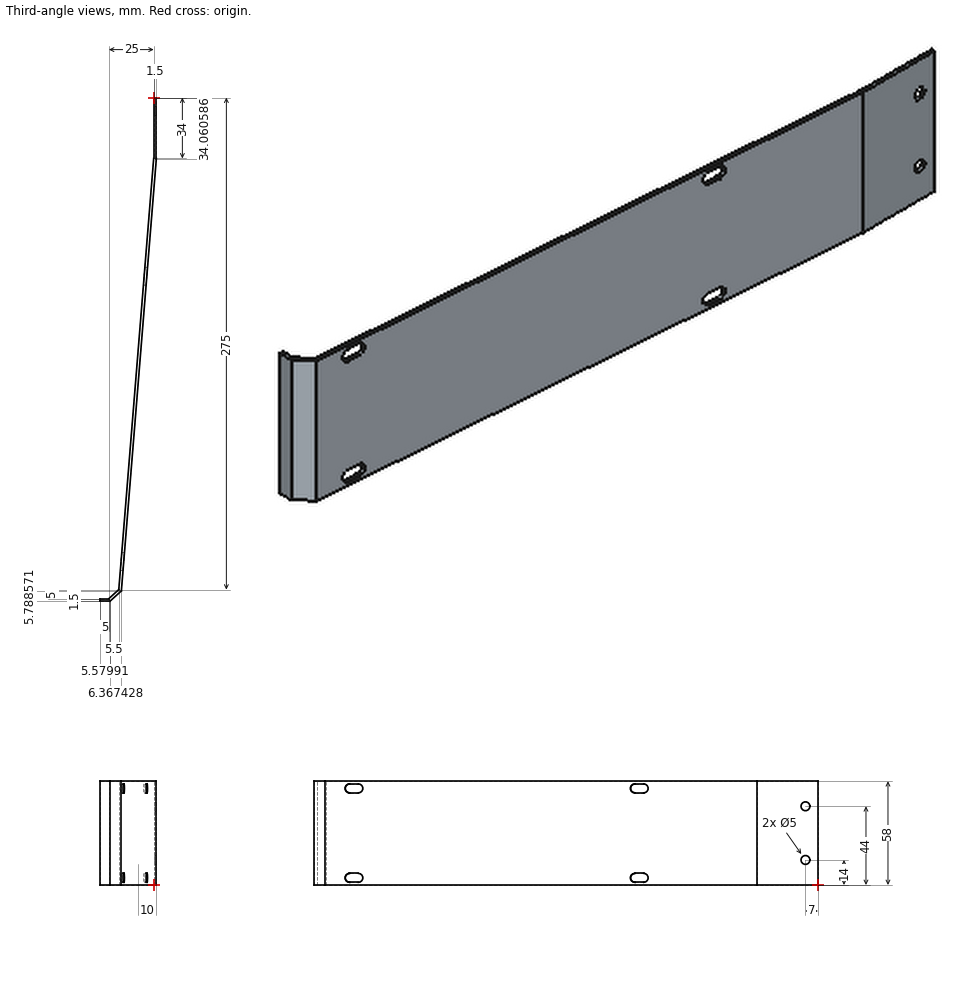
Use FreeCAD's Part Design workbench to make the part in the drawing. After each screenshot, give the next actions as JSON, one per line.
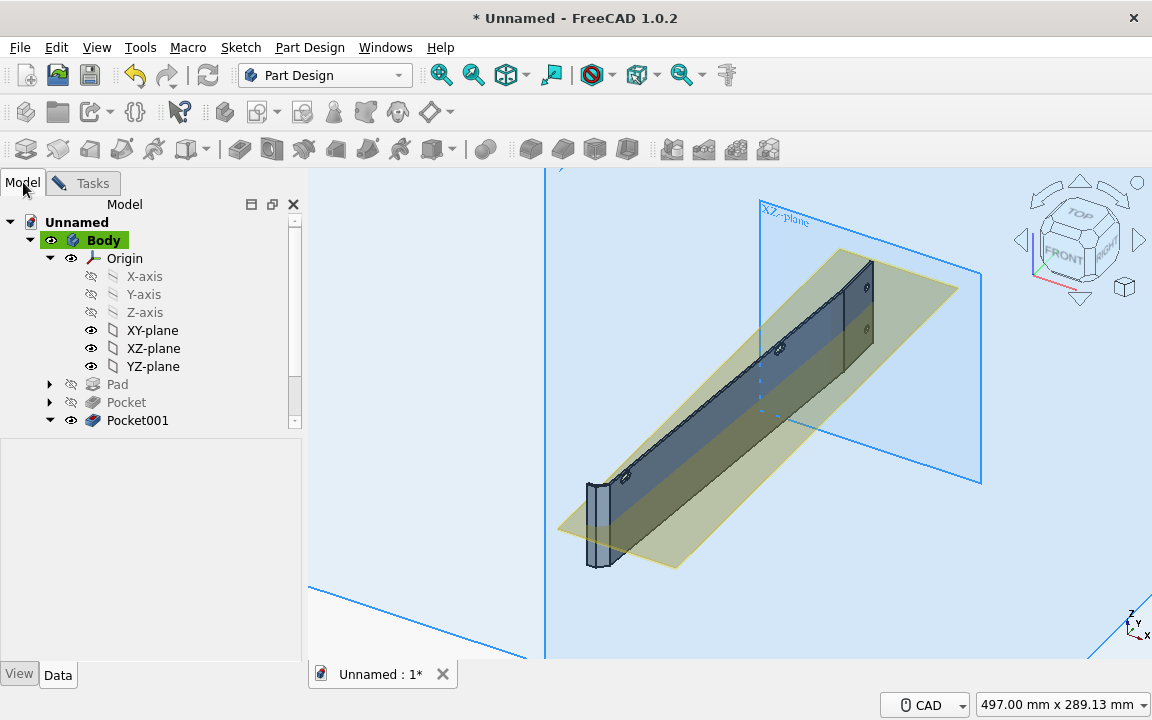
{"action": "scroll", "coordinate": [100, 326], "scroll_direction": "down", "scroll_amount": 3}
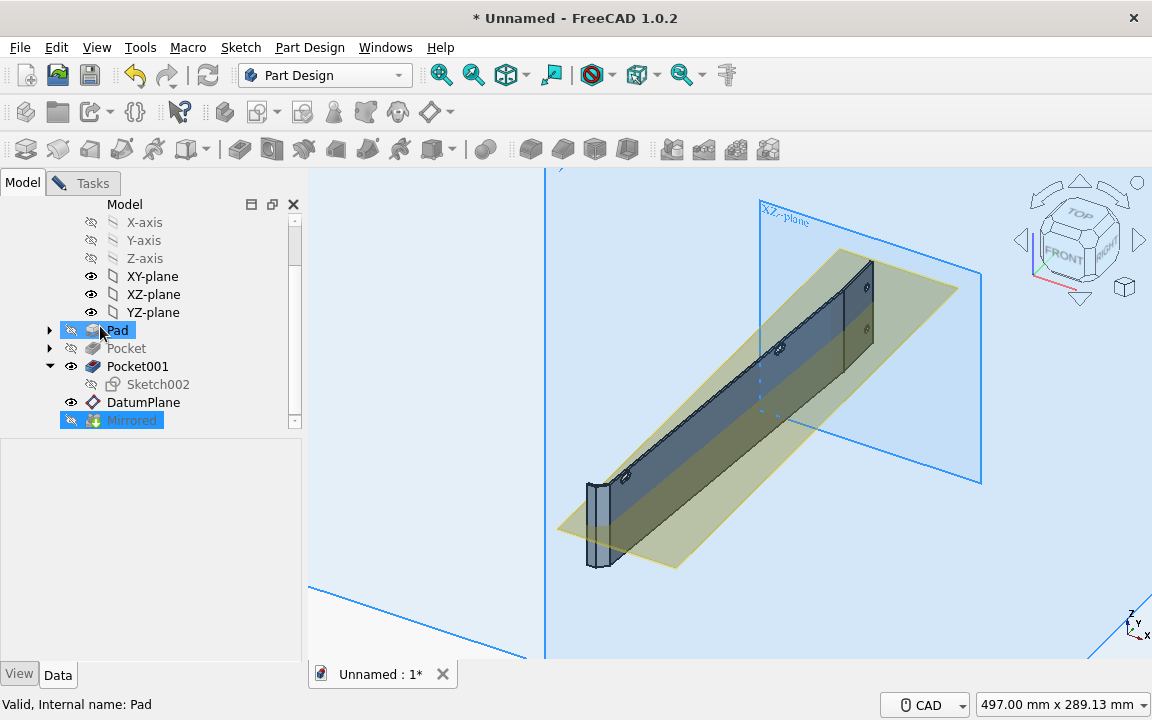
{"action": "left_click", "coordinate": [116, 402]}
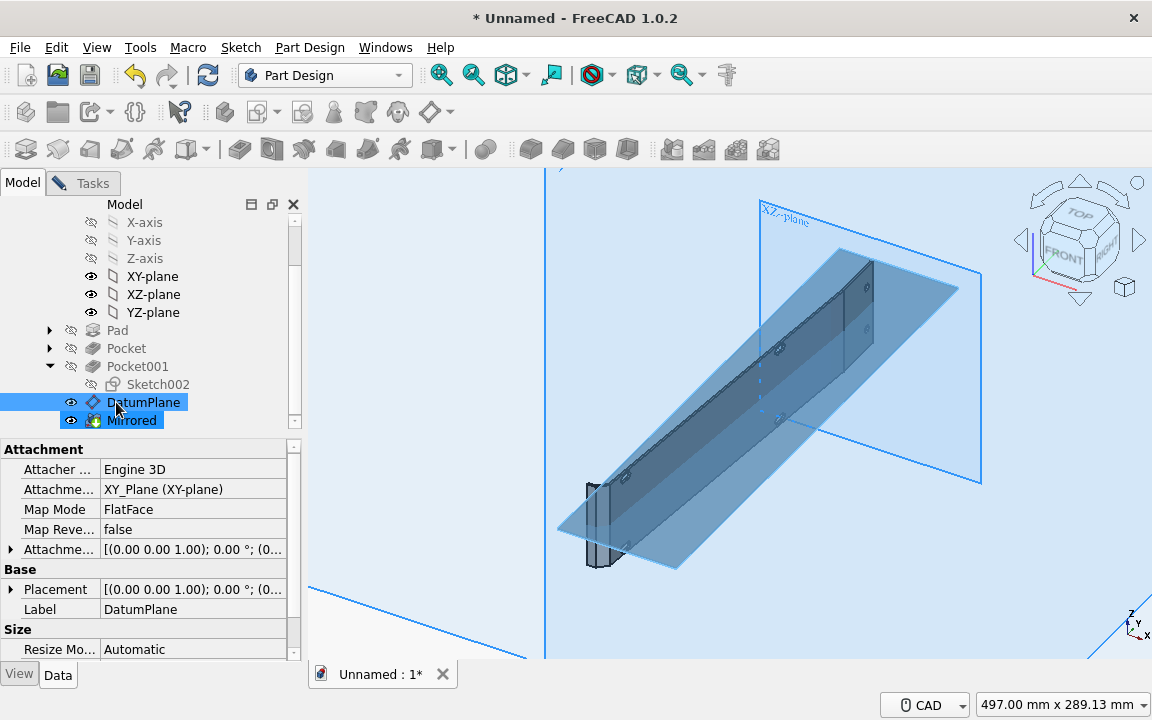
{"action": "left_click", "coordinate": [84, 182]}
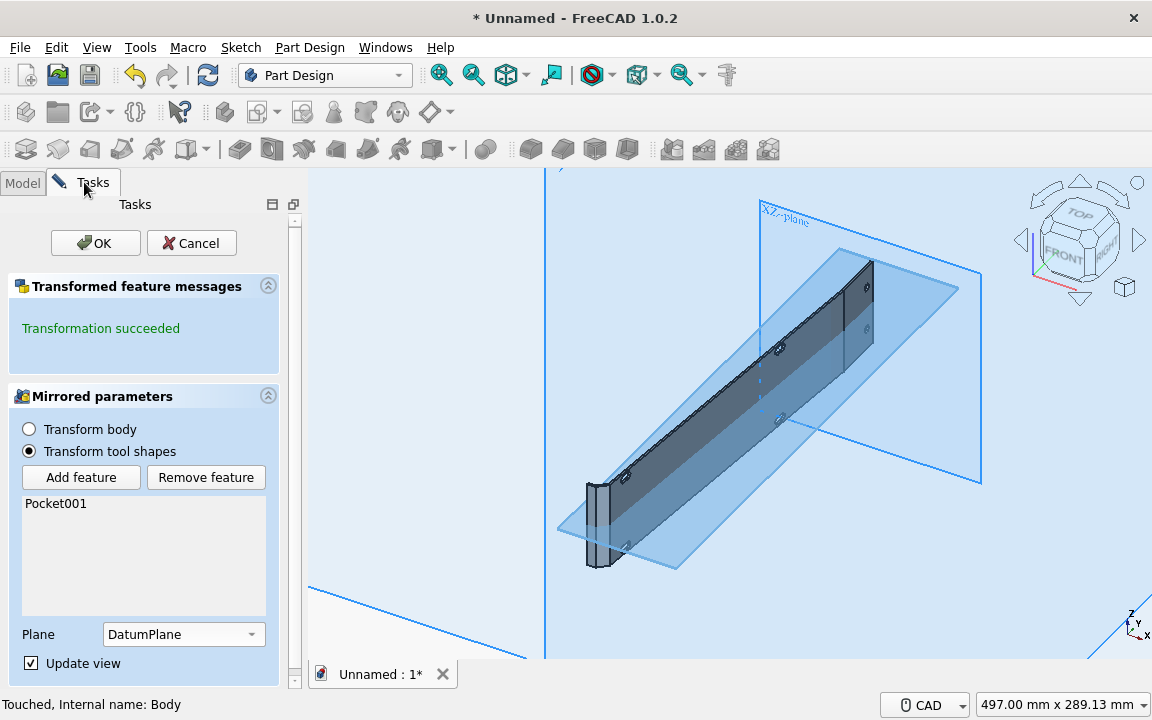
{"action": "left_click", "coordinate": [96, 243]}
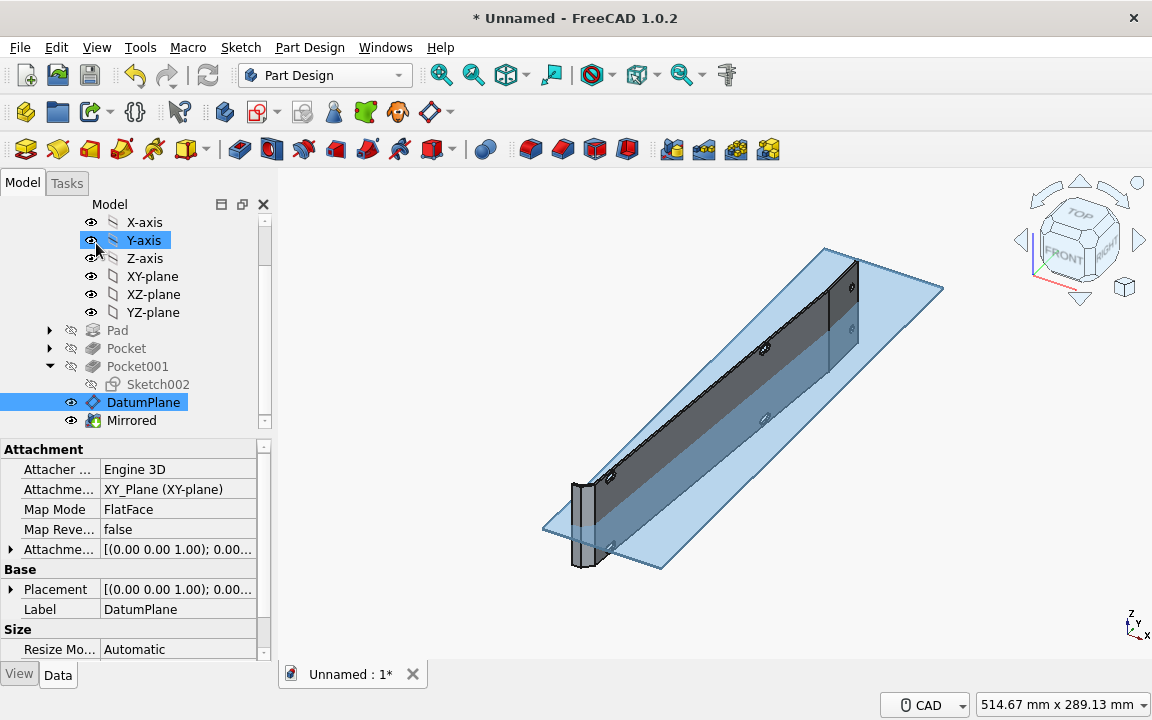
{"action": "left_click", "coordinate": [116, 402]}
{"action": "key", "text": "space"}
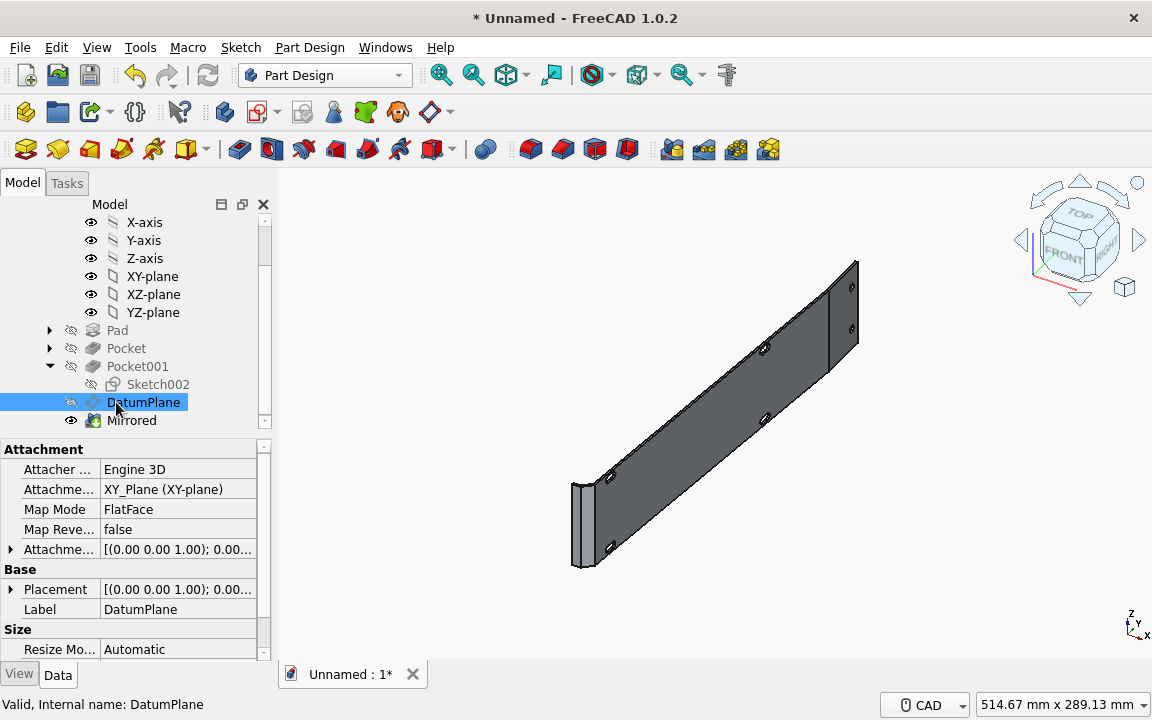
{"action": "key", "text": "0"}